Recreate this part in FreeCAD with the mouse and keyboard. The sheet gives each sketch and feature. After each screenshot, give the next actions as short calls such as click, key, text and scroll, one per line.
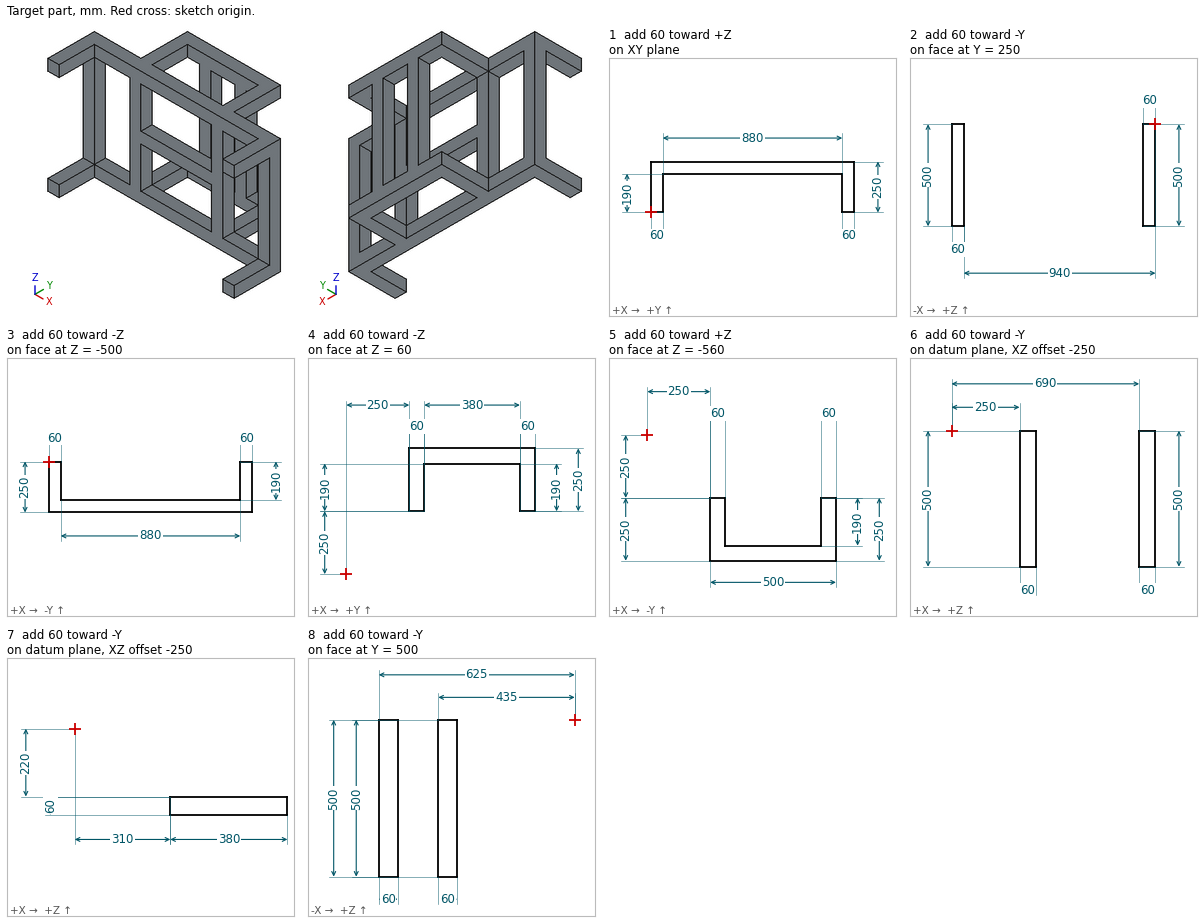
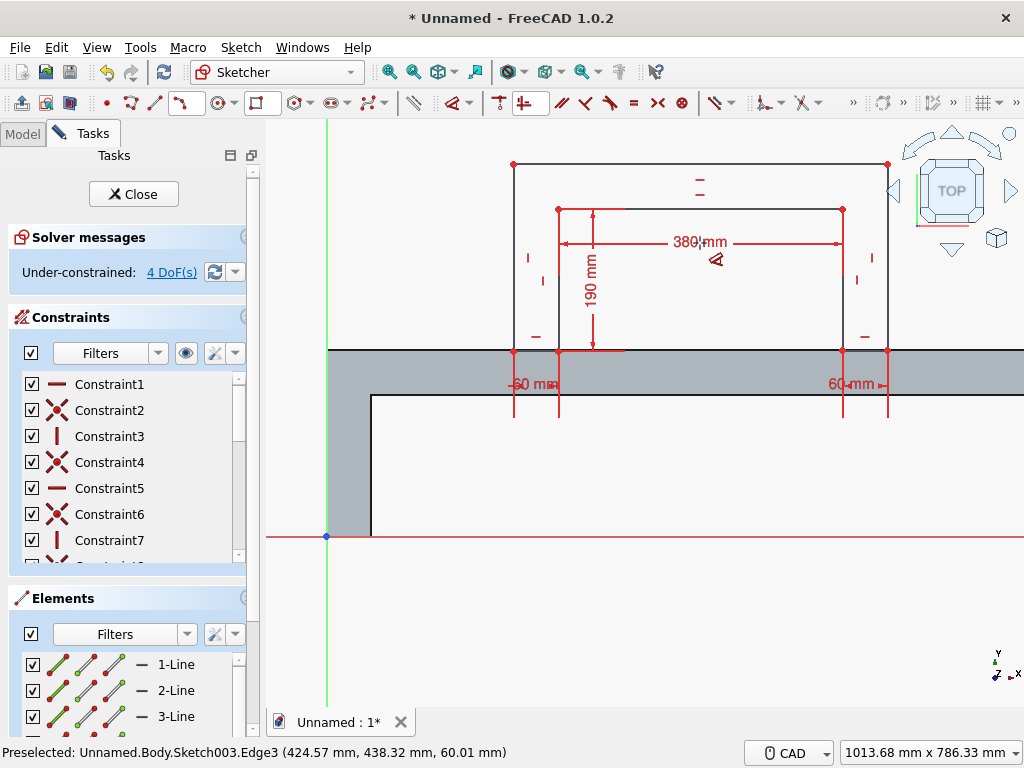
click(843, 252)
click(809, 280)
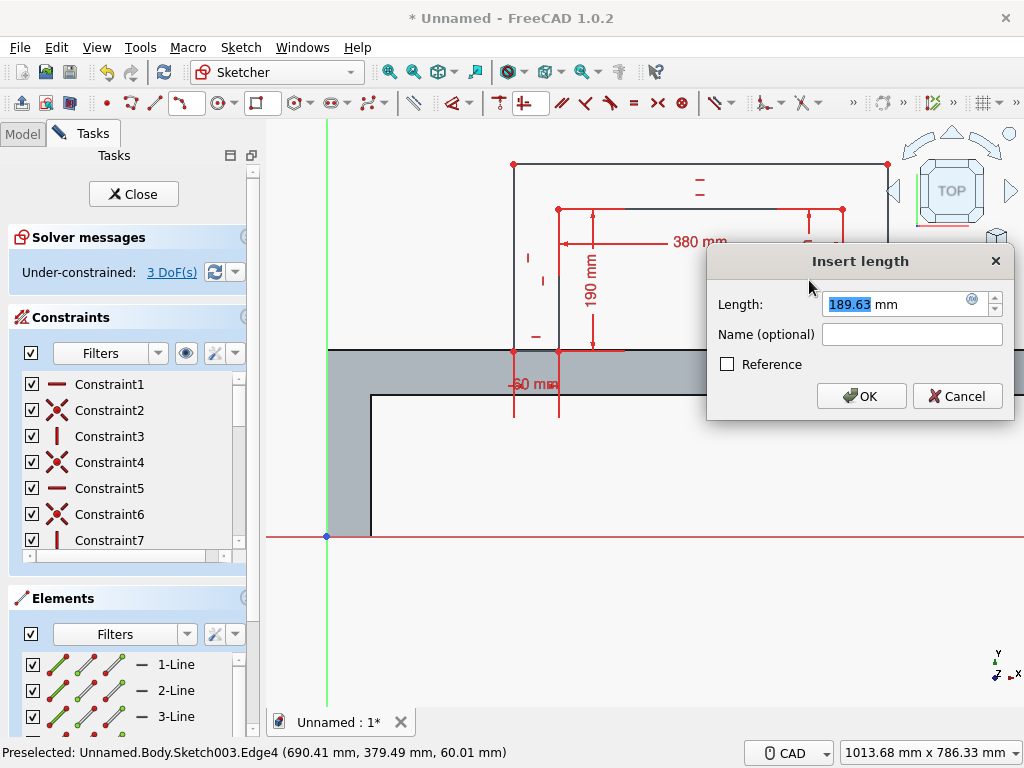
text(190)
key(Return)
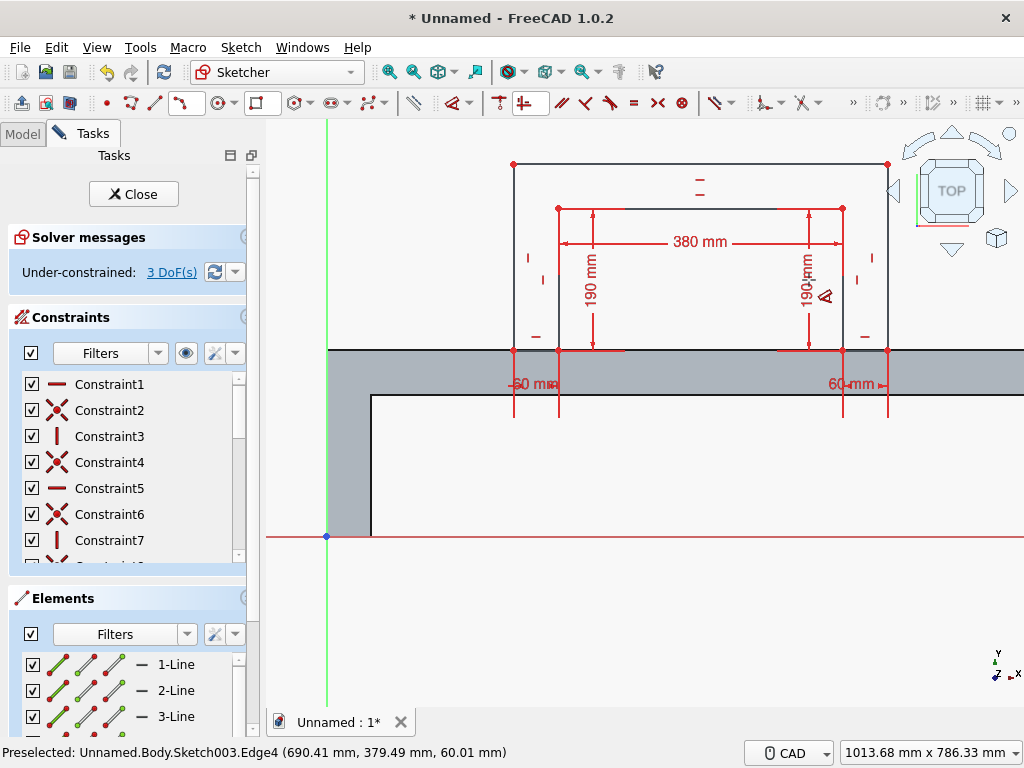
scroll(515, 541, down, 2)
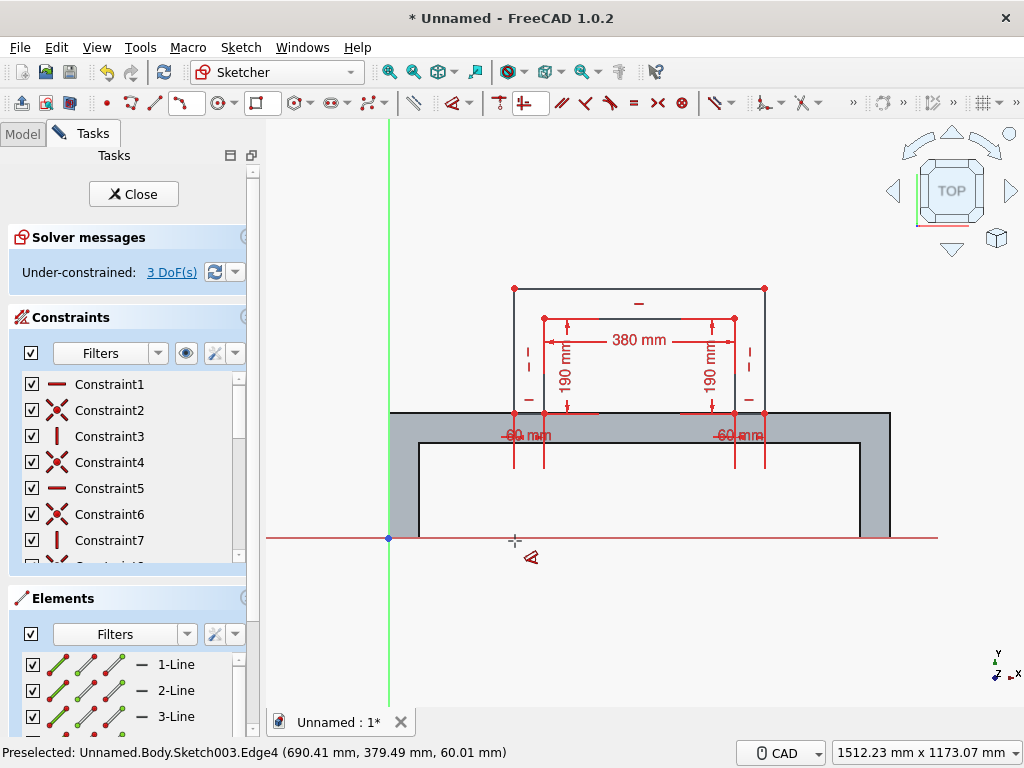
click(765, 376)
click(799, 351)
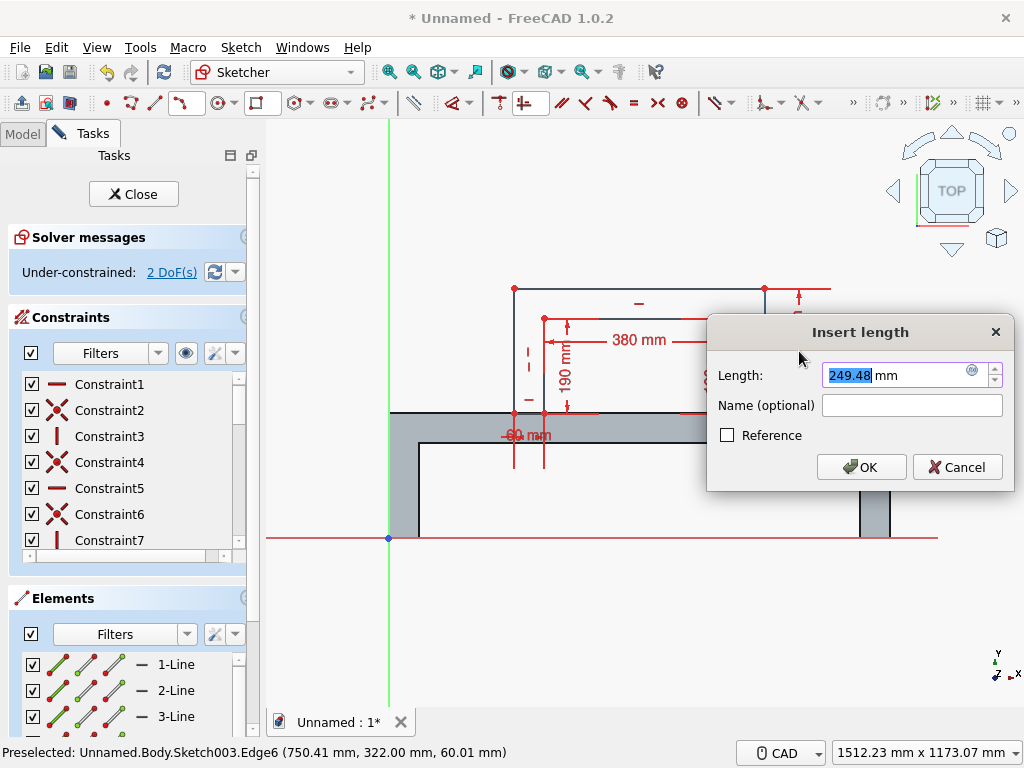
text(250)
key(Return)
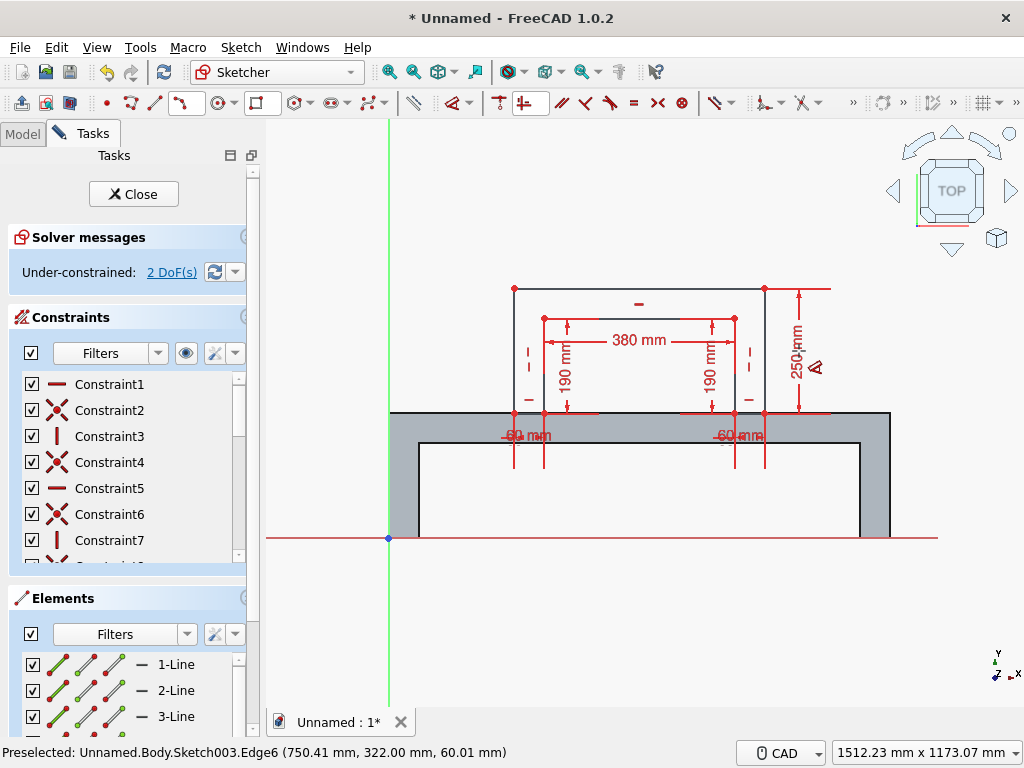
click(514, 414)
click(452, 572)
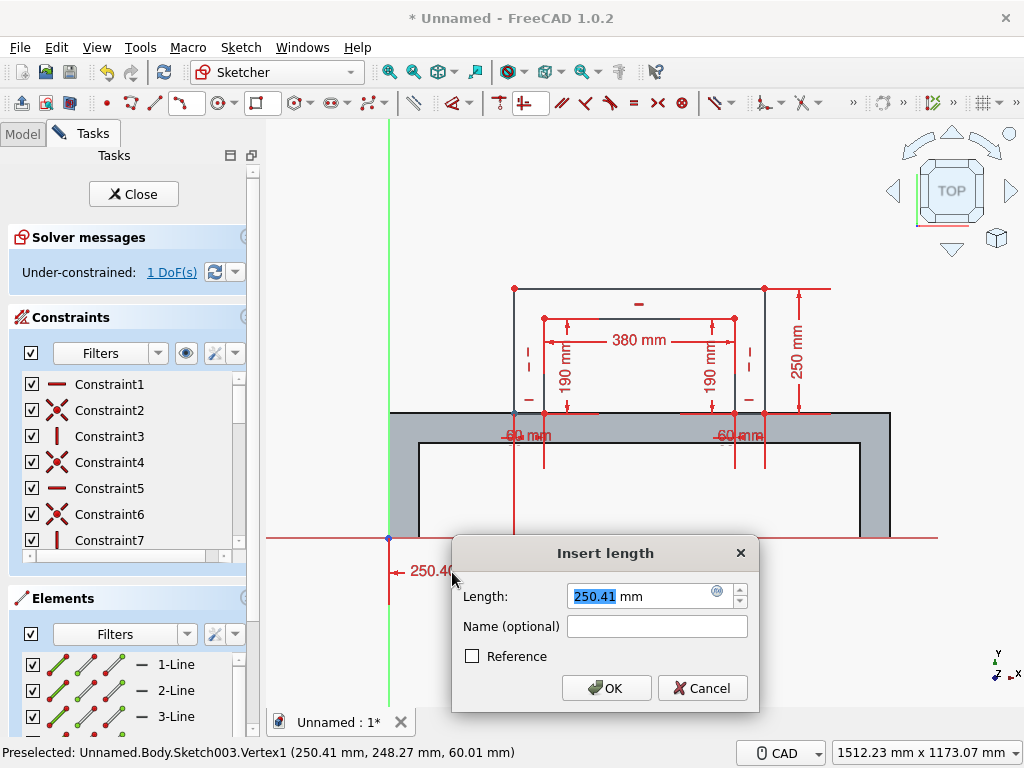
text(250)
key(Return)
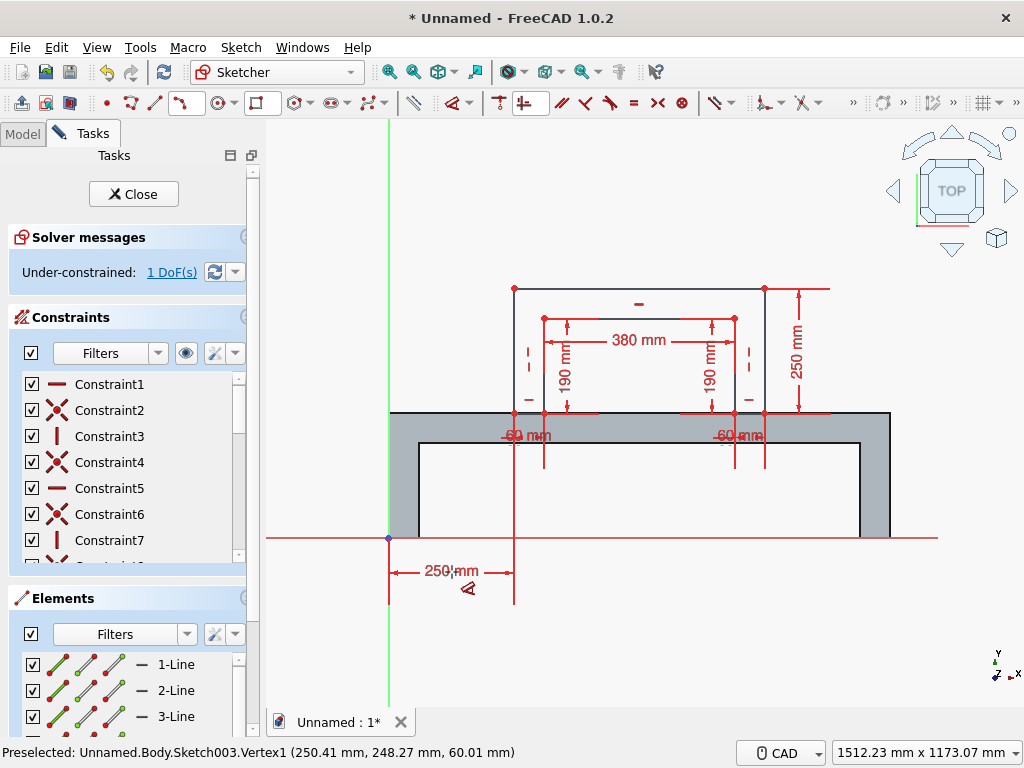
click(514, 414)
click(355, 476)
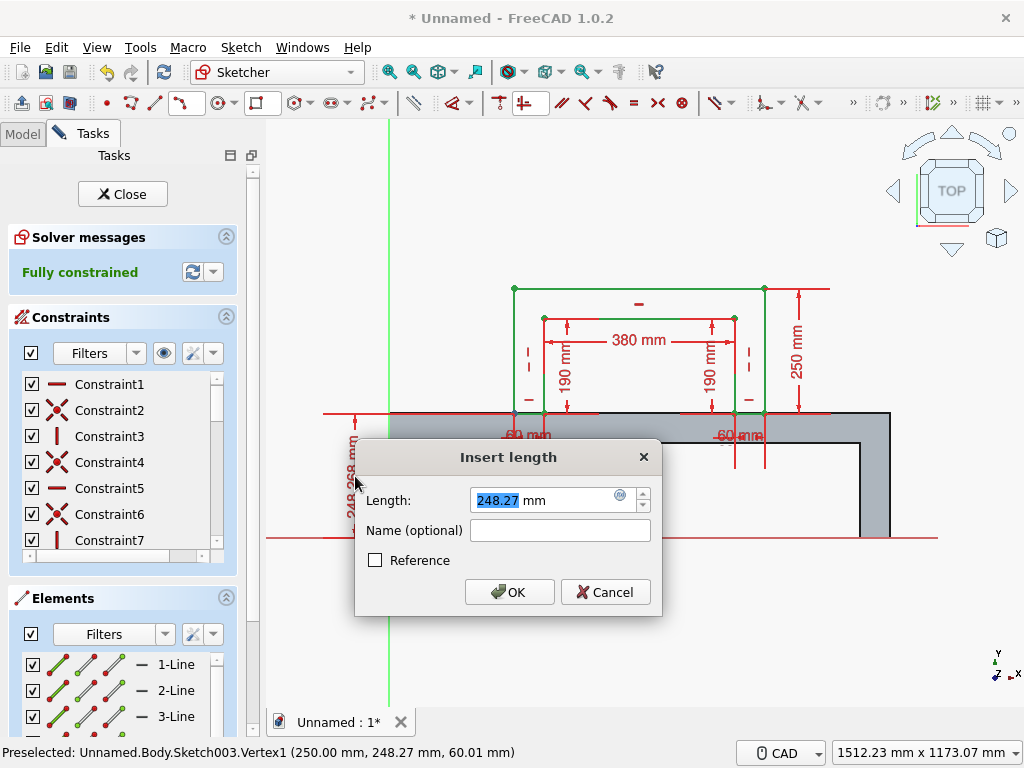
text(250)
key(Return)
key(Escape)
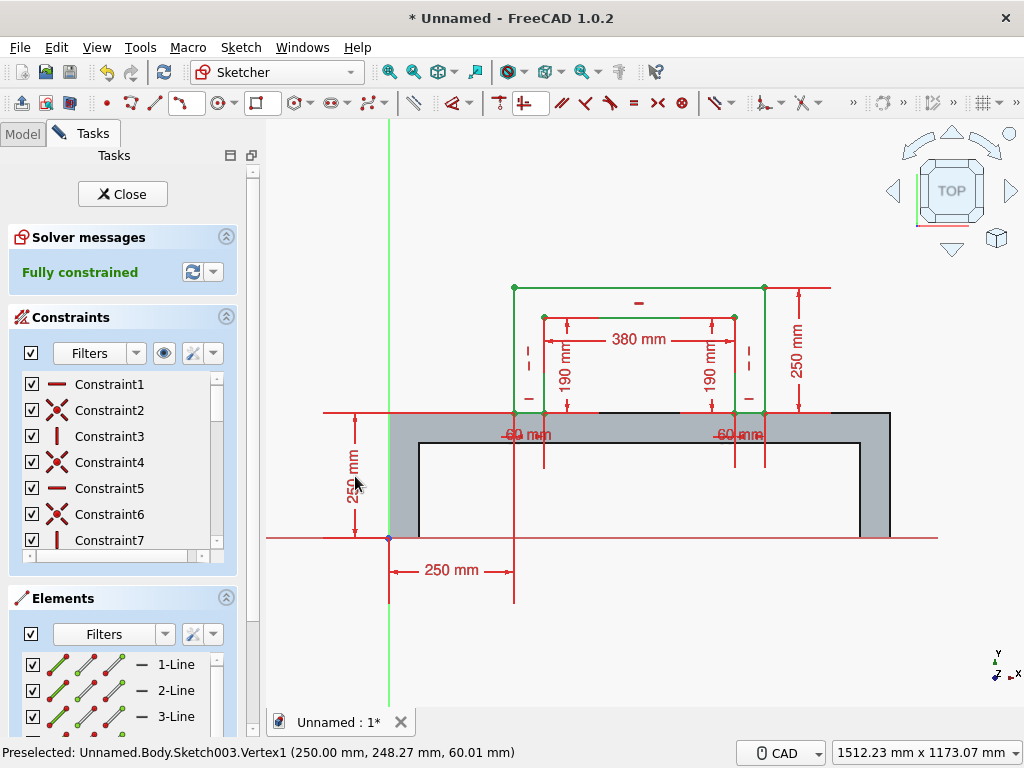
click(123, 194)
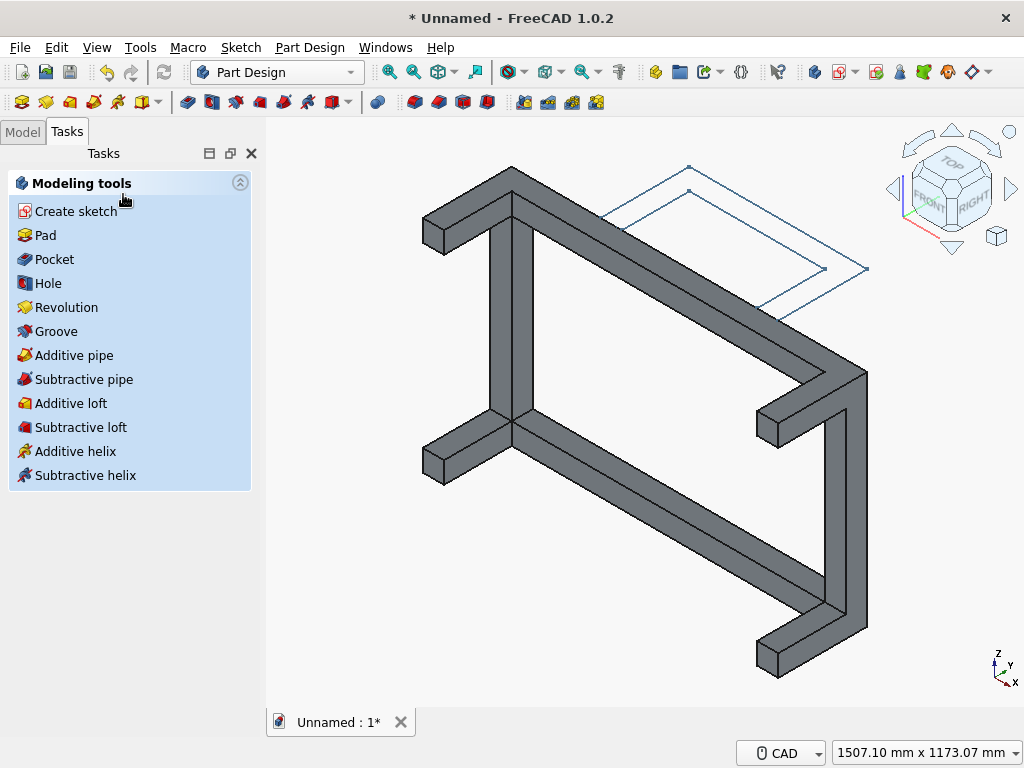
click(22, 102)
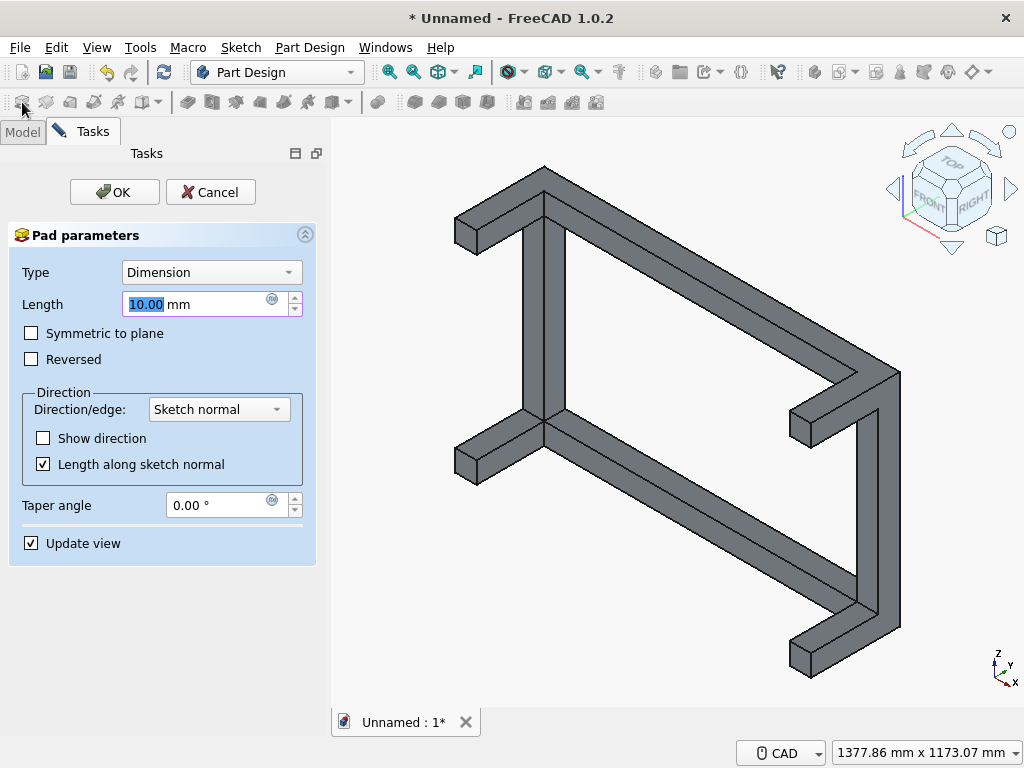
text(60)
key(Tab)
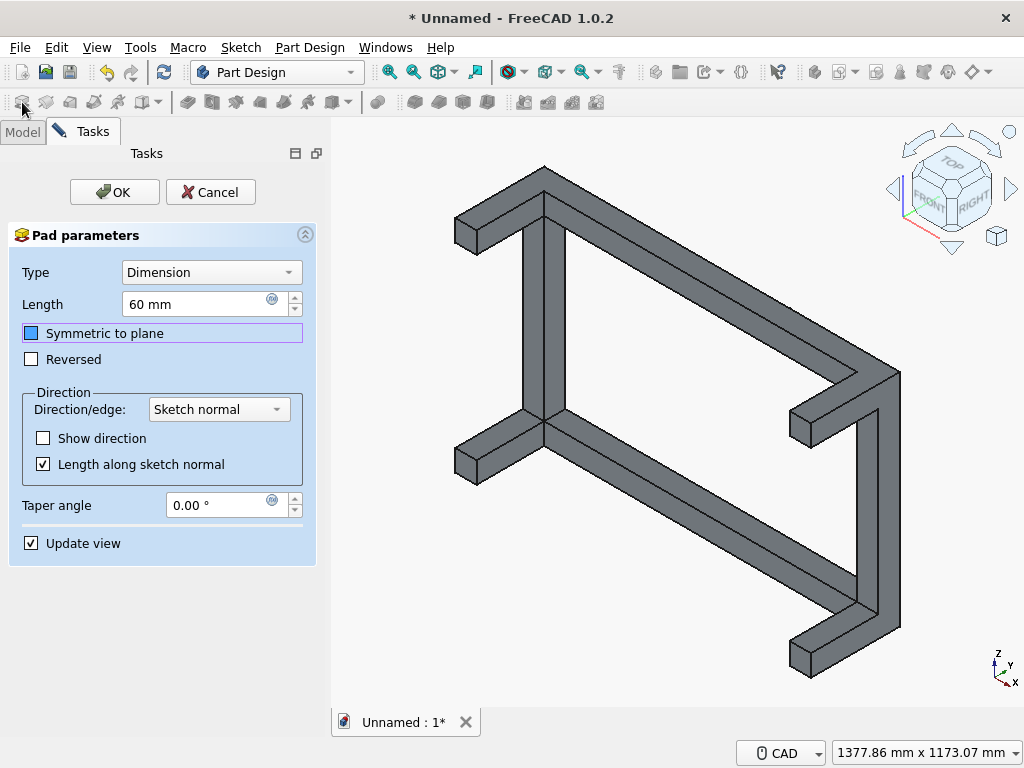
click(30, 359)